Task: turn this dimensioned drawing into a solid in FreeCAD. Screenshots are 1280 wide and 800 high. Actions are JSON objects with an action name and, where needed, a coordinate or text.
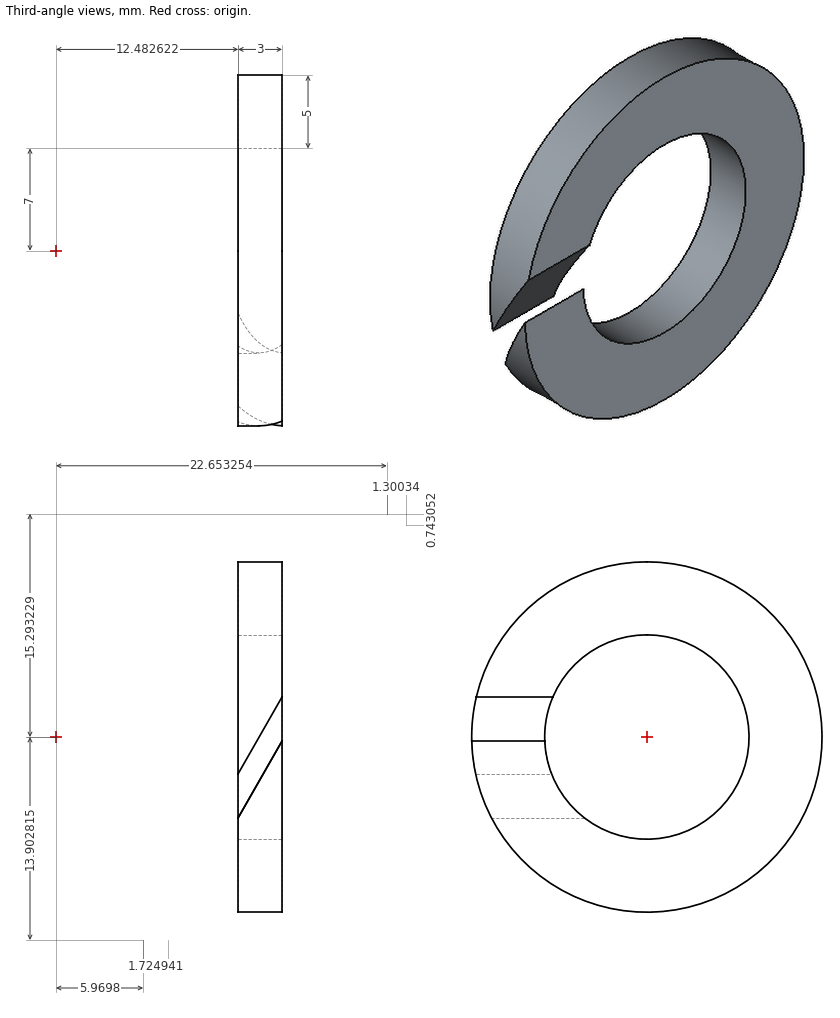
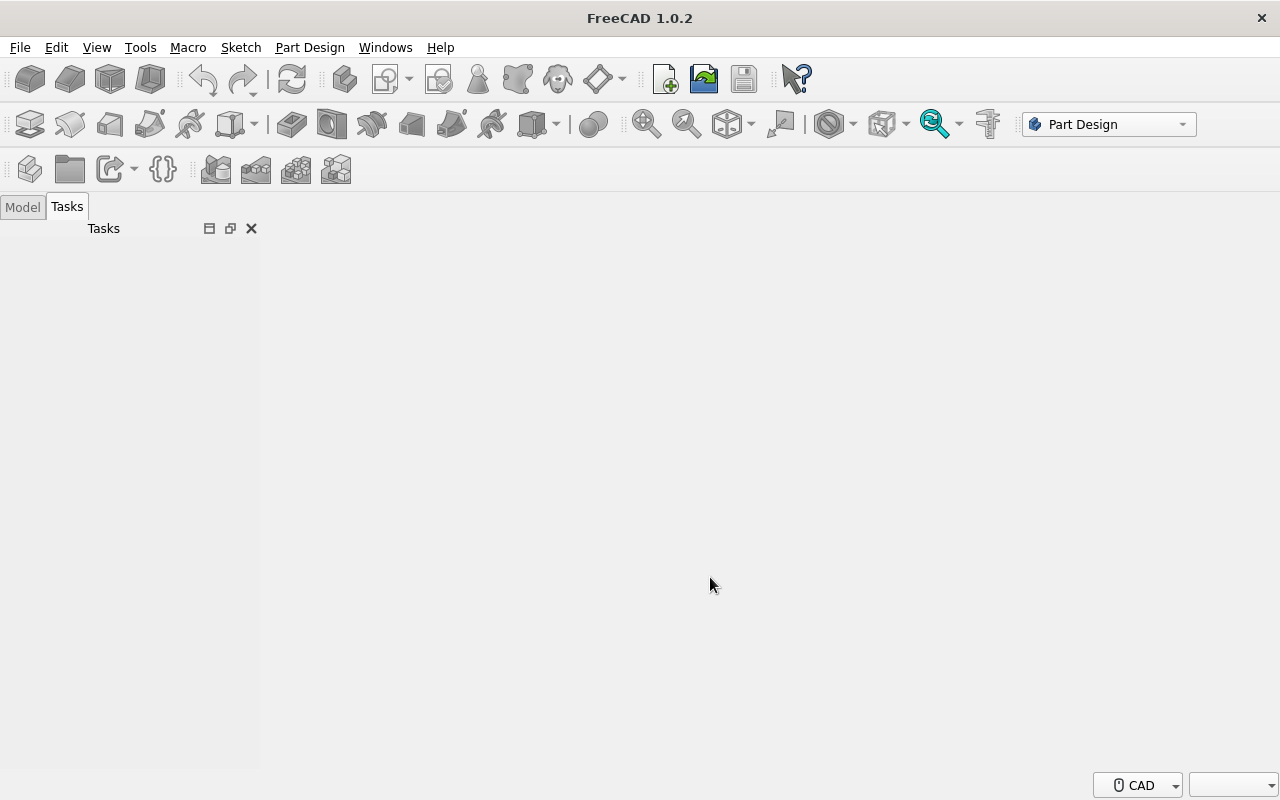
{"action": "key", "text": "ctrl+n"}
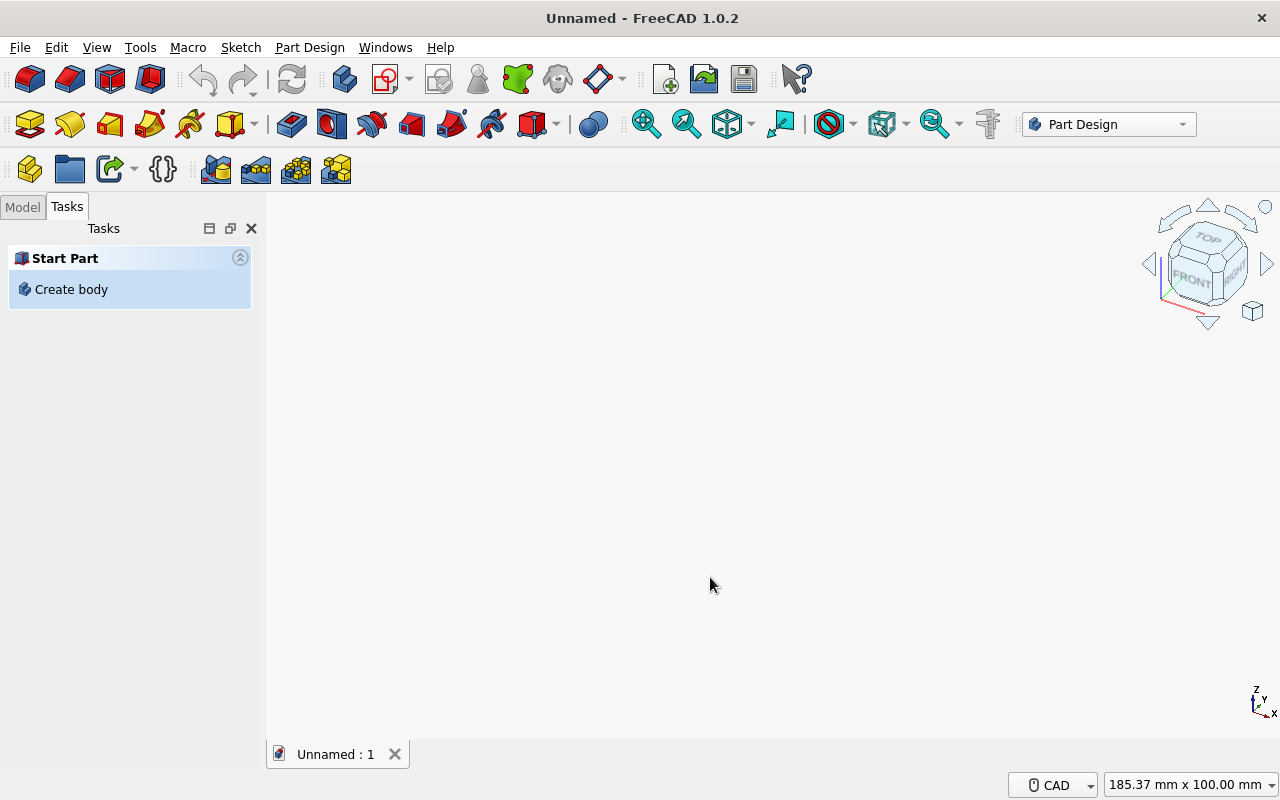
{"action": "left_click", "coordinate": [386, 80]}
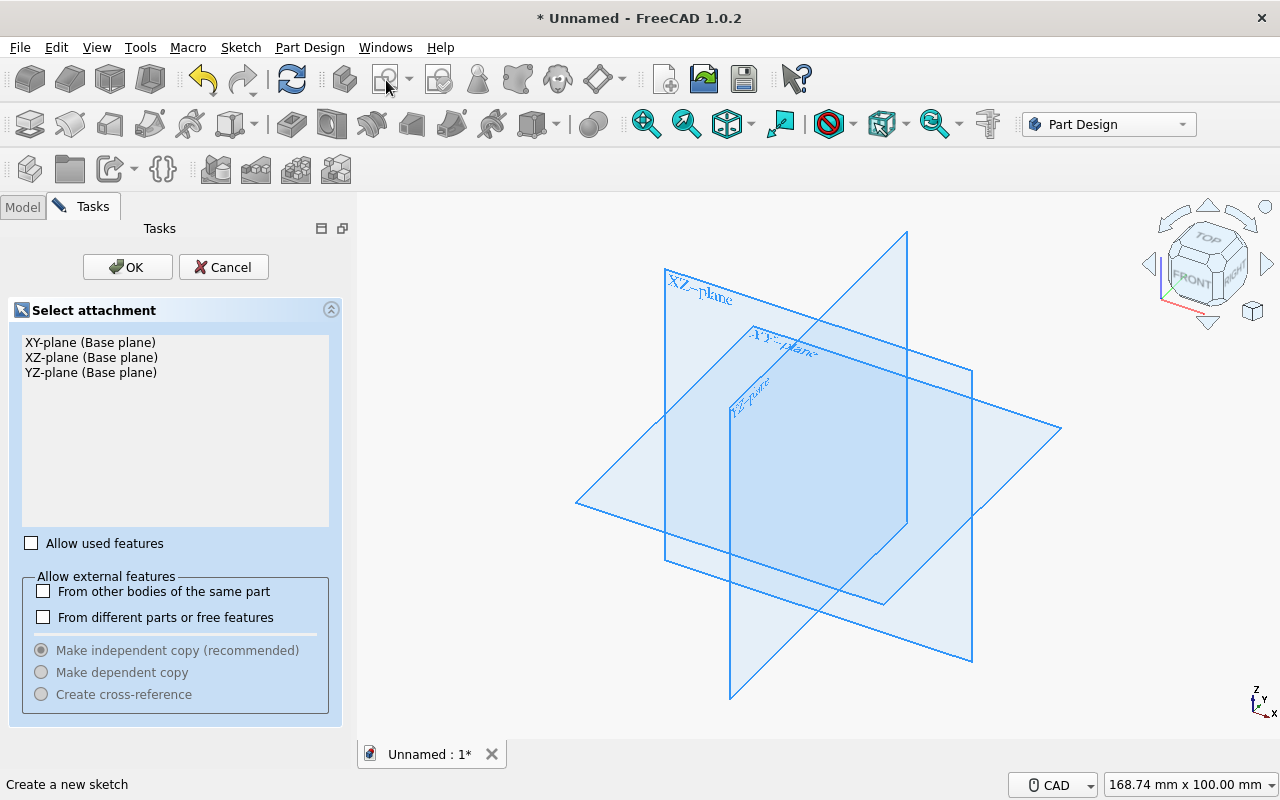
{"action": "left_click", "coordinate": [82, 342]}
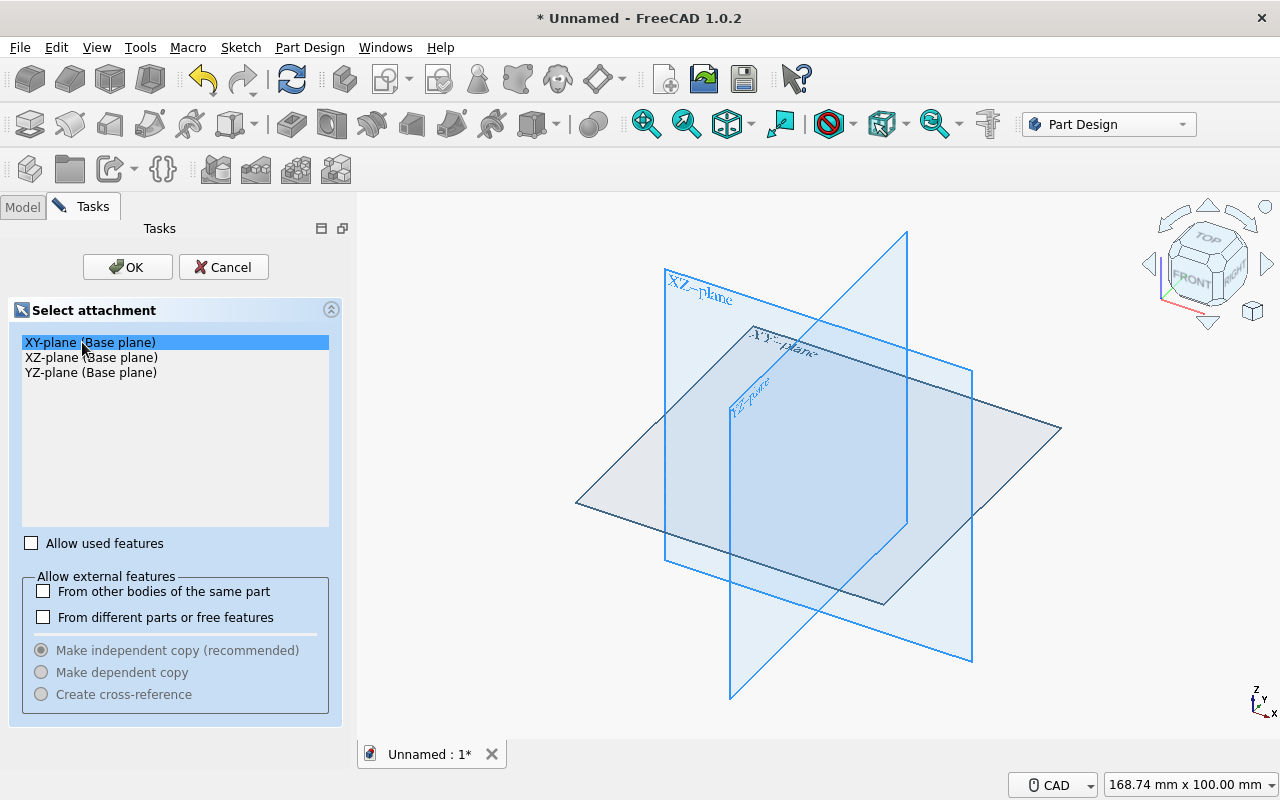
{"action": "left_click", "coordinate": [128, 267]}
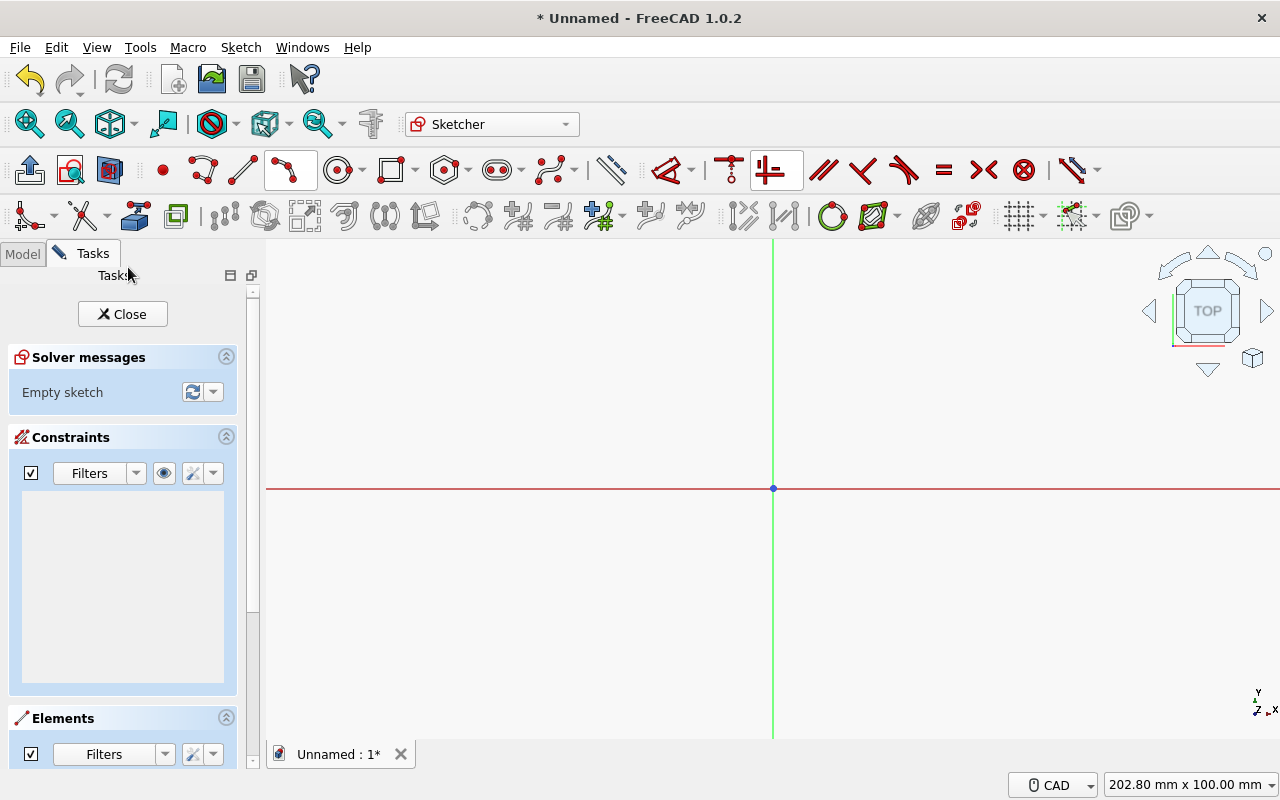
{"action": "scroll", "coordinate": [854, 438], "scroll_direction": "up", "scroll_amount": 13}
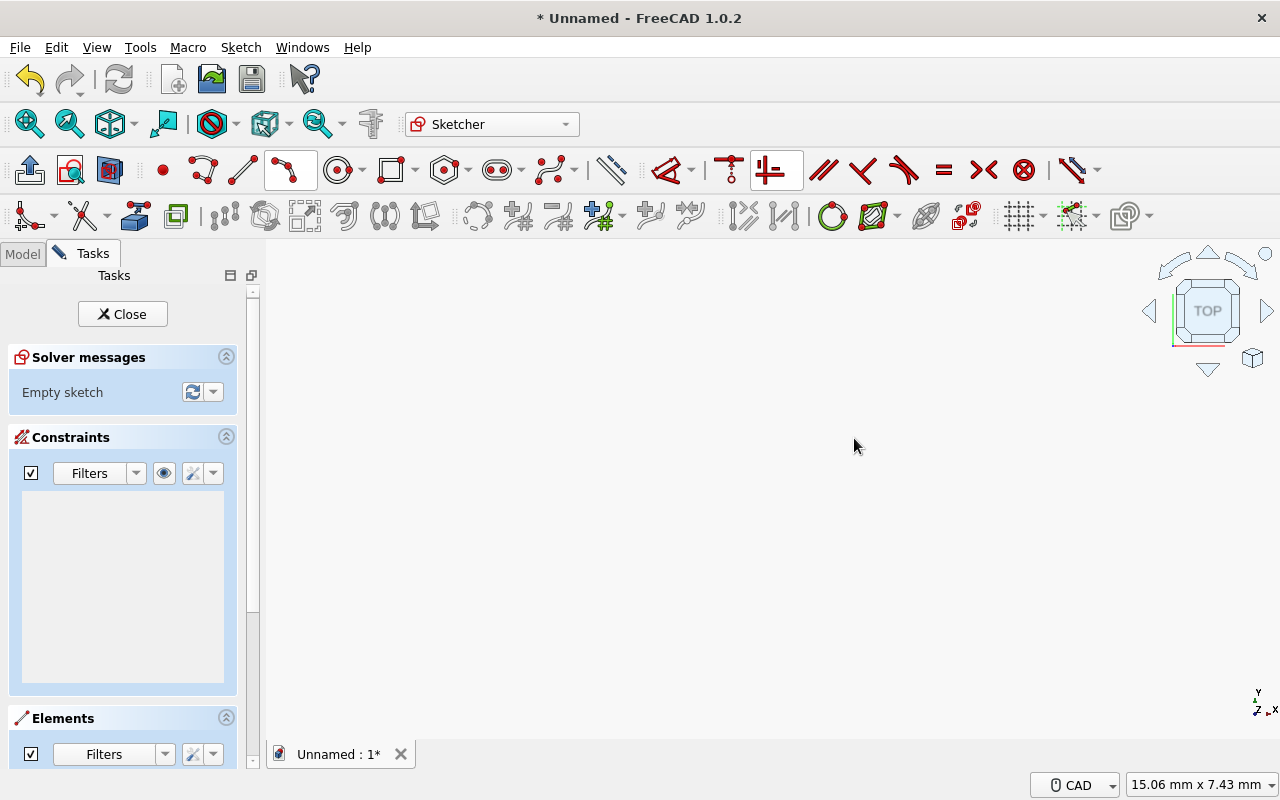
{"action": "left_click", "coordinate": [392, 170]}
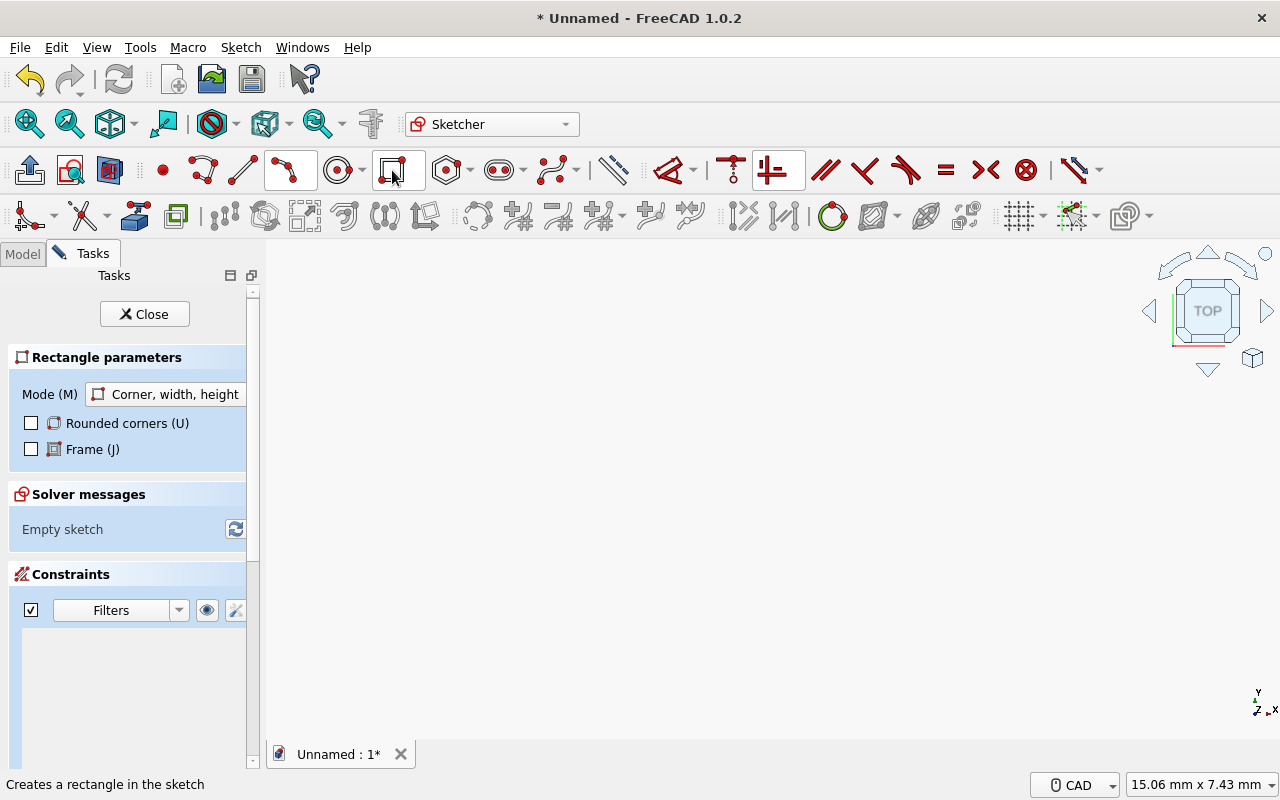
{"action": "left_click", "coordinate": [597, 312]}
{"action": "mouse_move", "coordinate": [798, 648]}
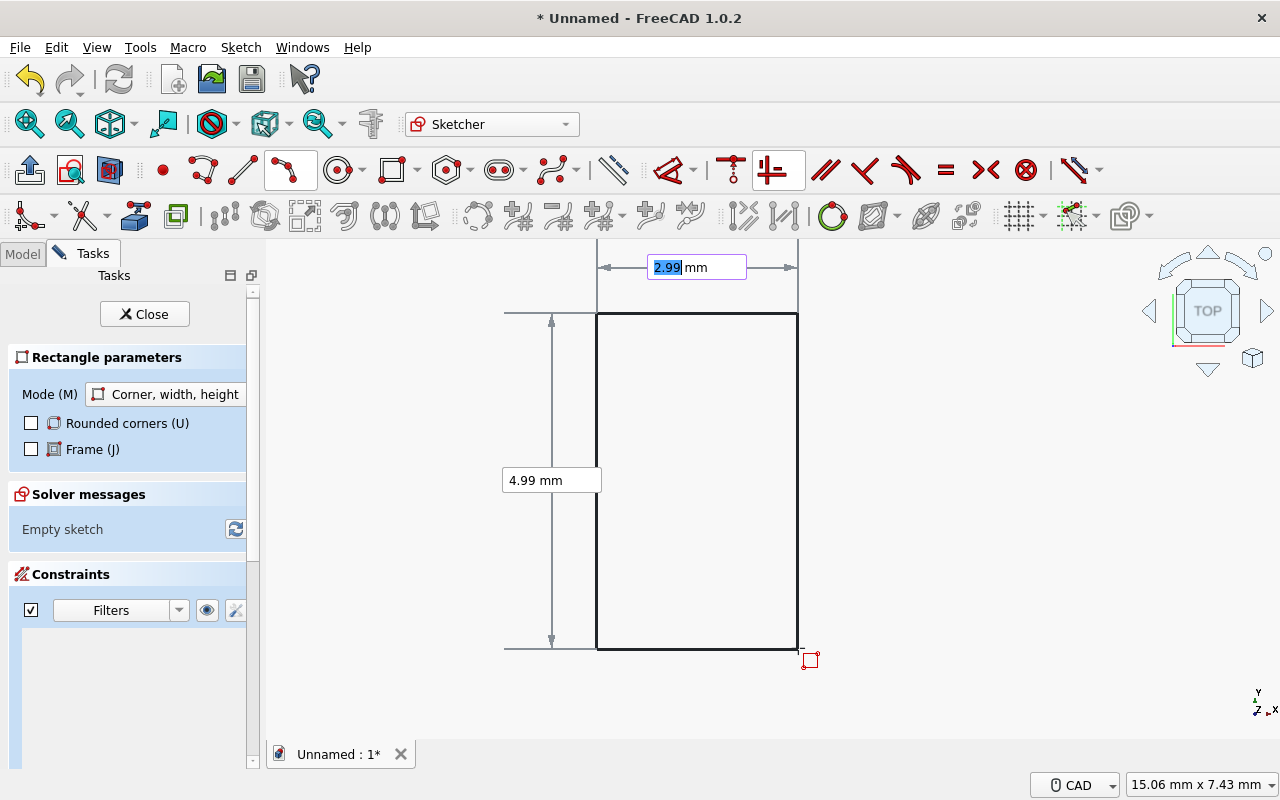
{"action": "type", "text": "3"}
{"action": "key", "text": "Tab"}
{"action": "type", "text": "5"}
{"action": "key", "text": "Return"}
{"action": "key", "text": "Escape"}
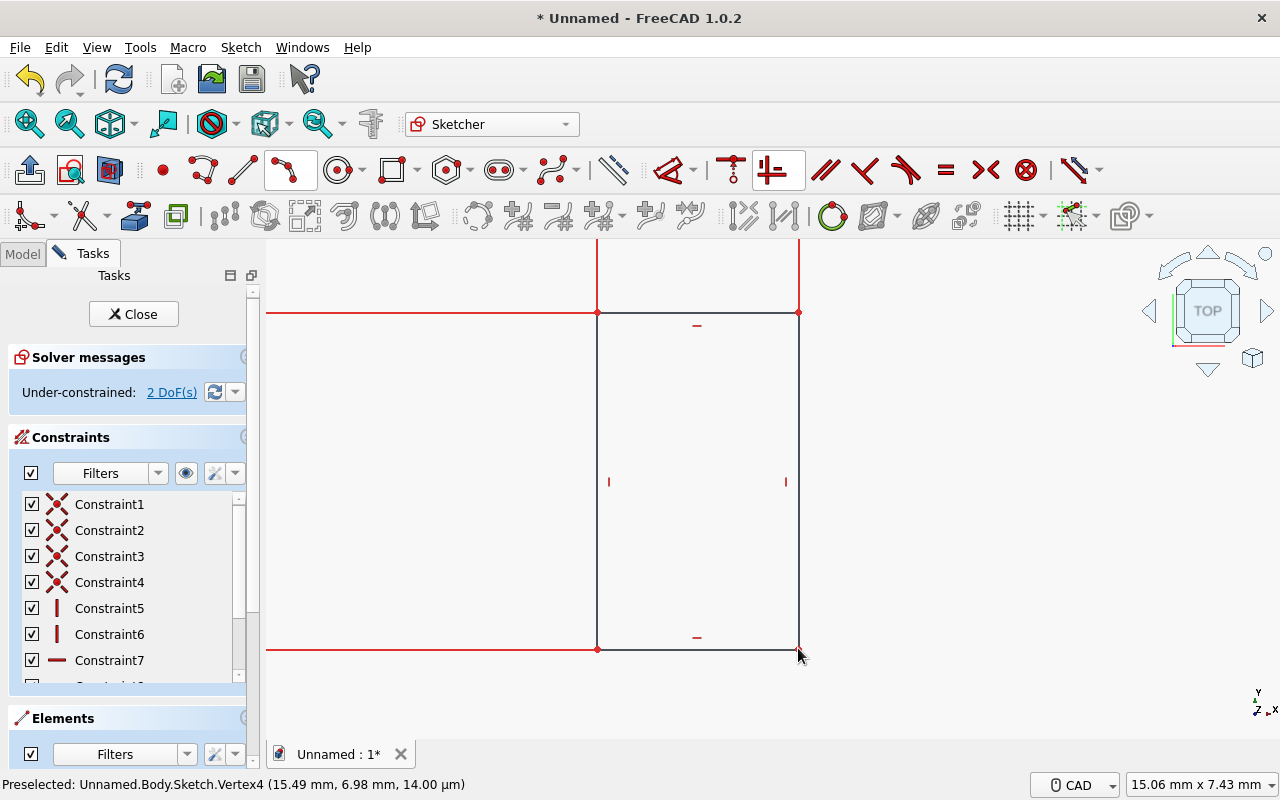
{"action": "key", "text": "d"}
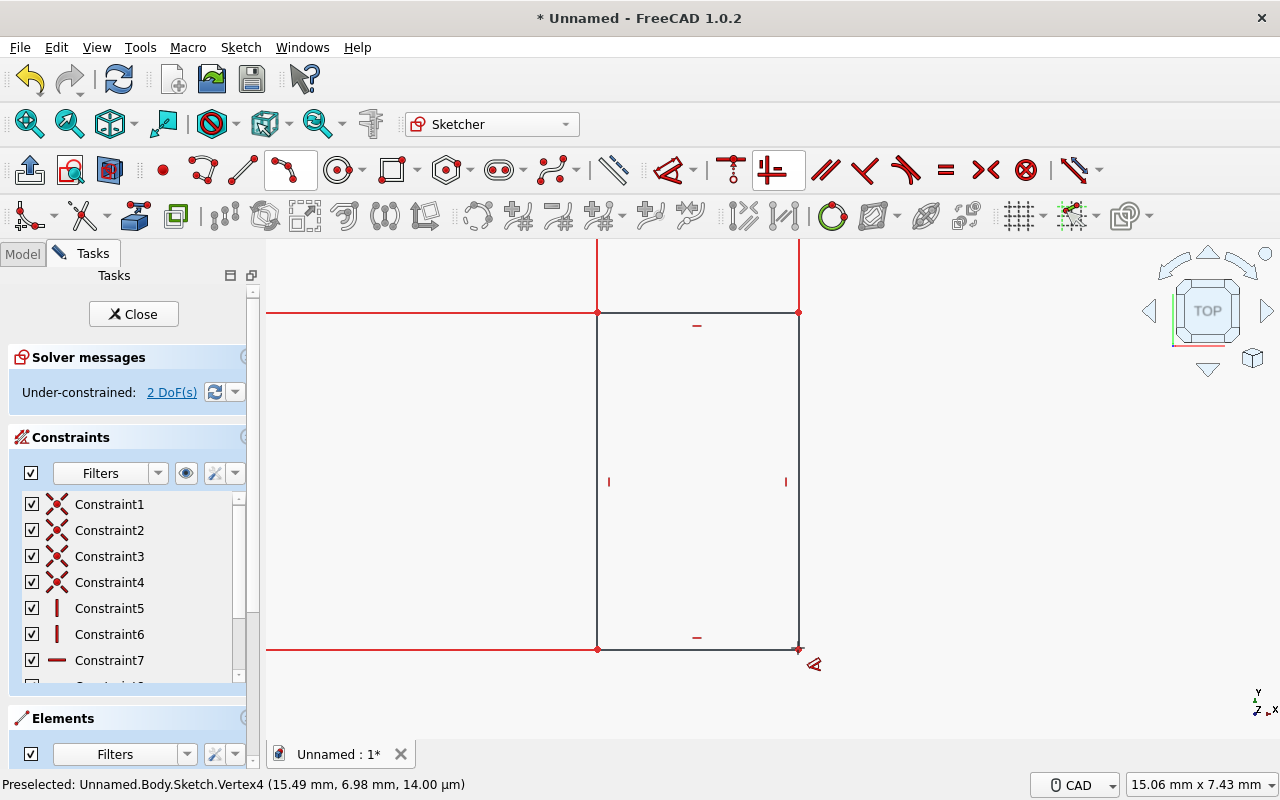
{"action": "left_click", "coordinate": [597, 650]}
{"action": "left_click", "coordinate": [631, 680]}